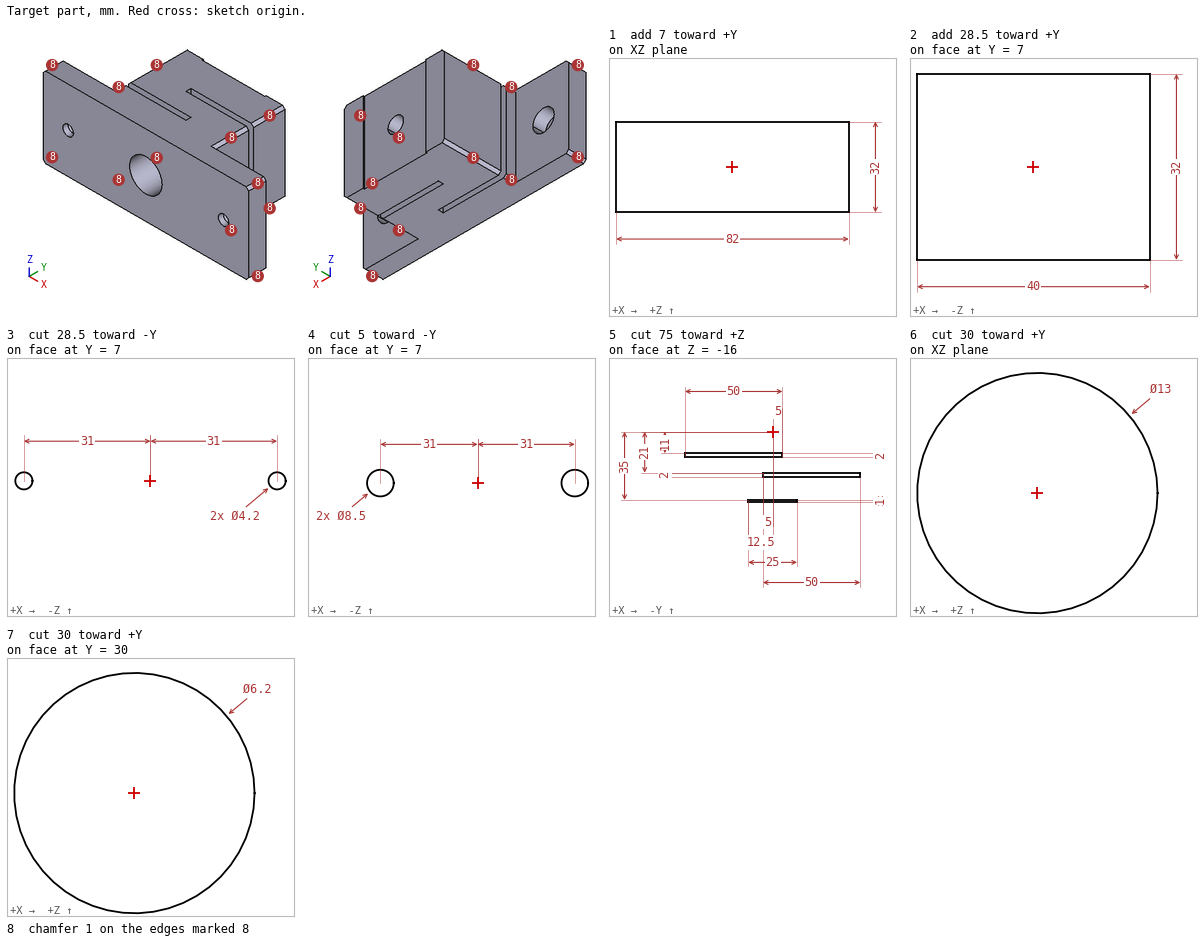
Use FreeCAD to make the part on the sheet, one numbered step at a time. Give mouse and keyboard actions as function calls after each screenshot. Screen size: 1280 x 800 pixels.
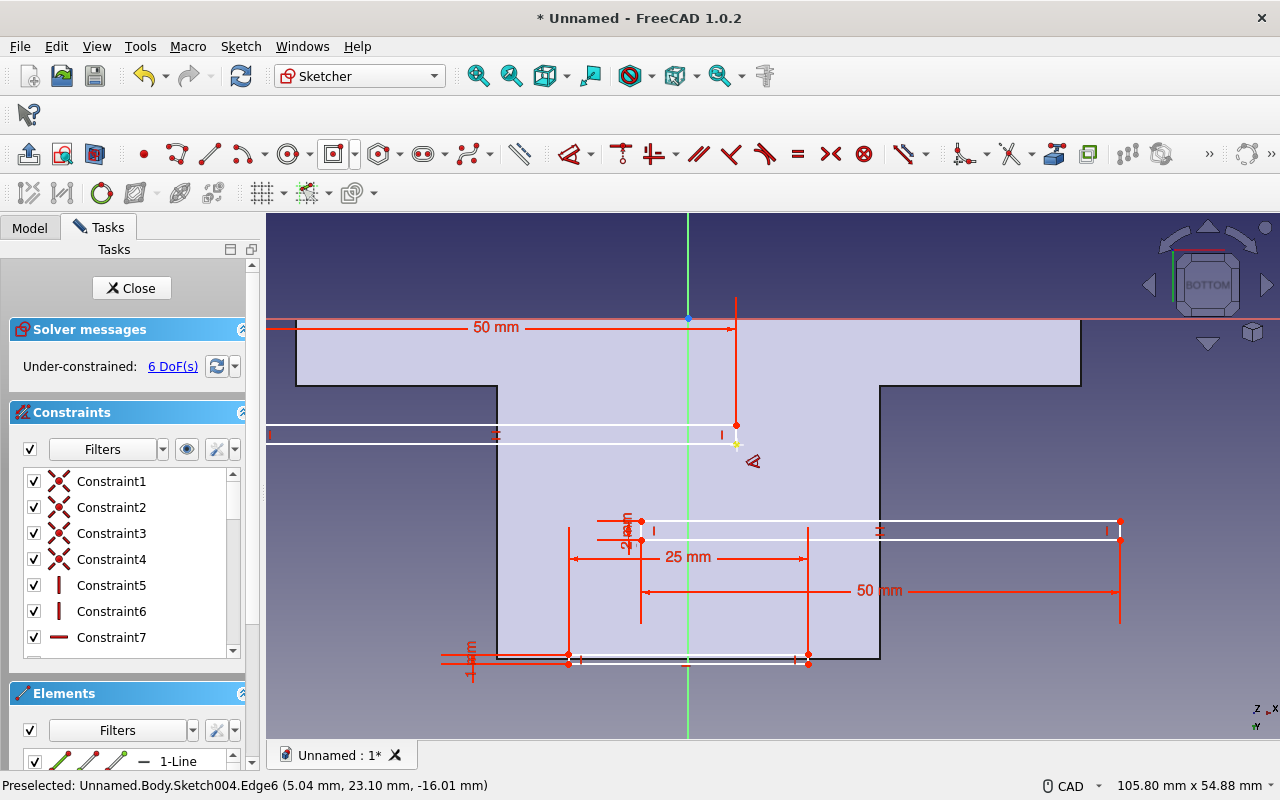
click(736, 444)
click(712, 285)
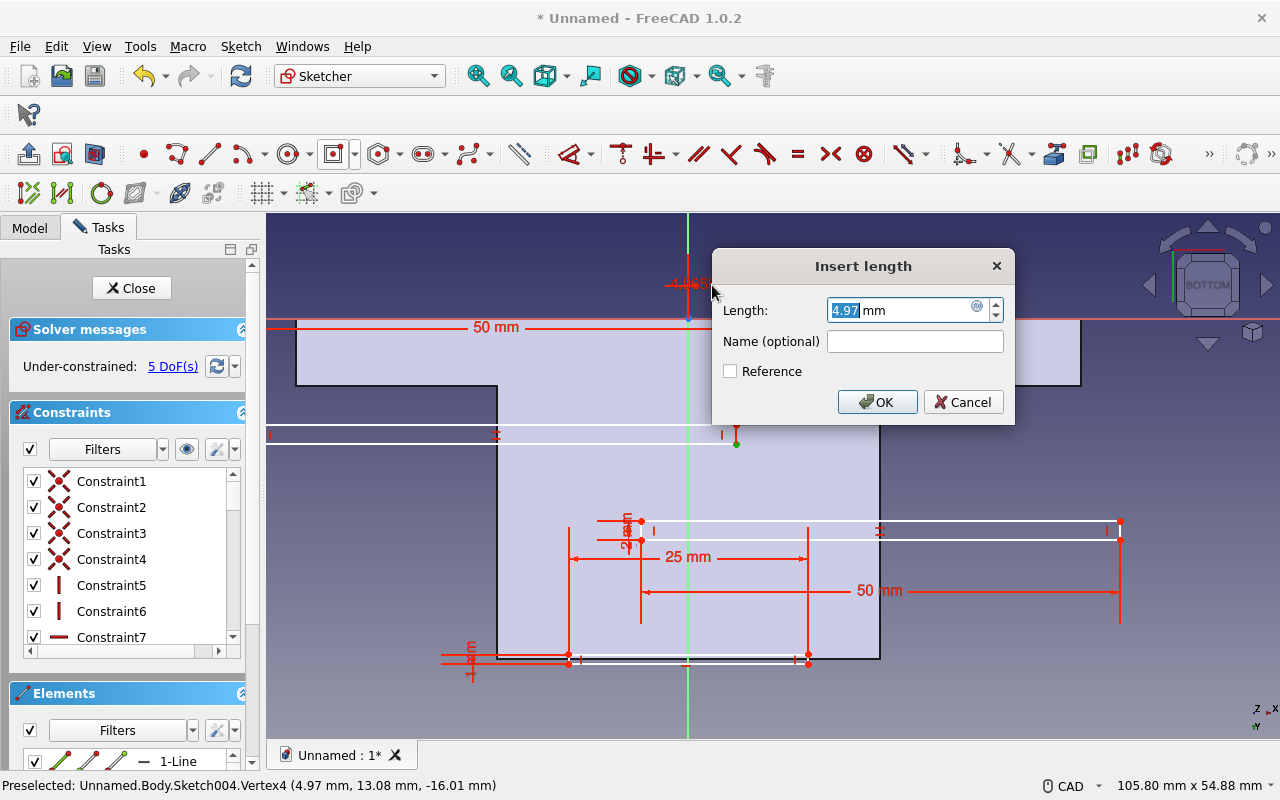
text(5)
key(Return)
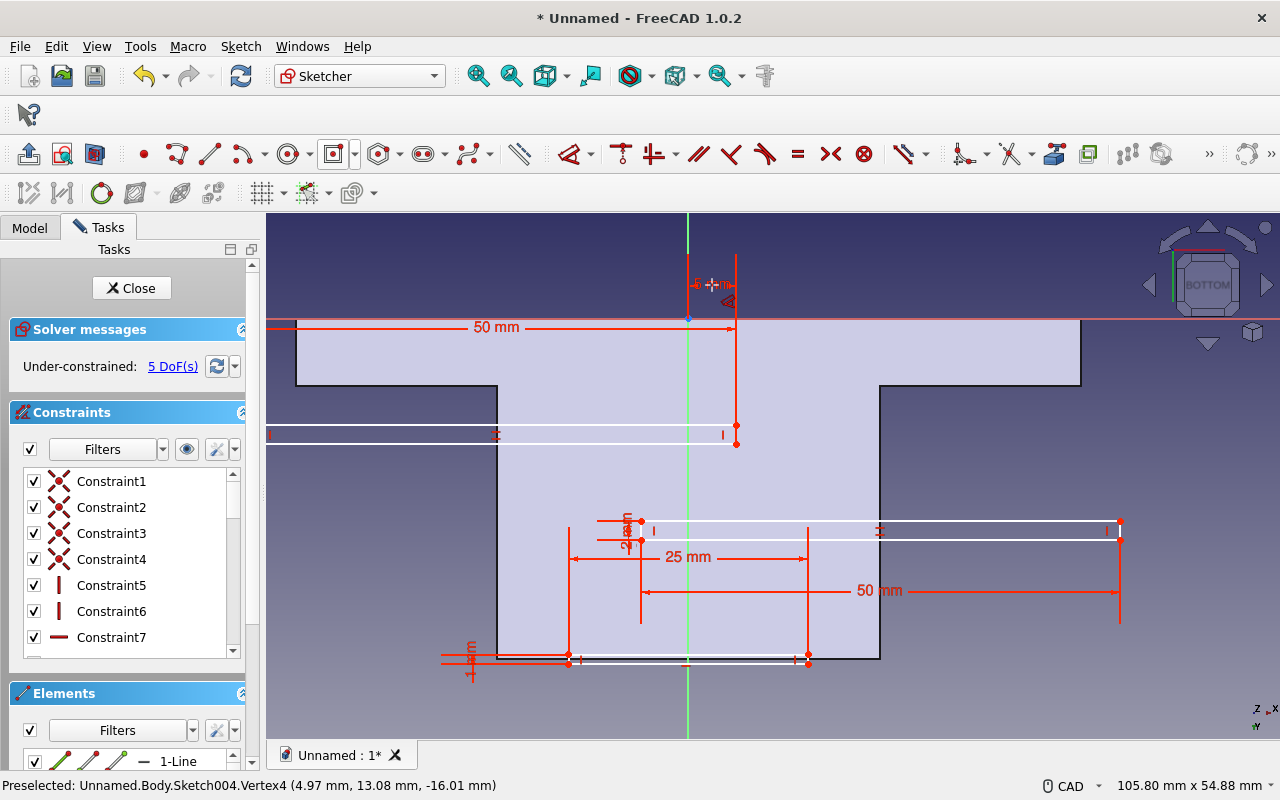
click(641, 521)
click(665, 555)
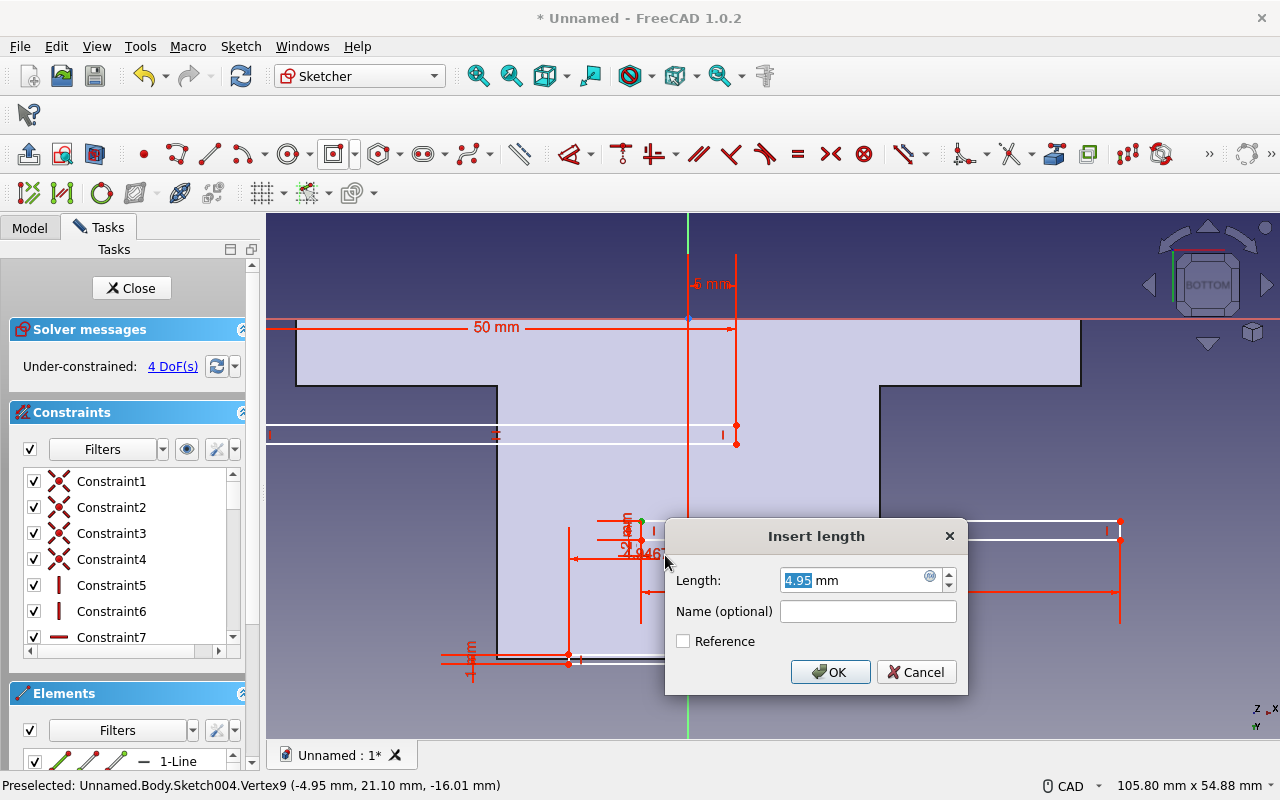
text(5)
key(Return)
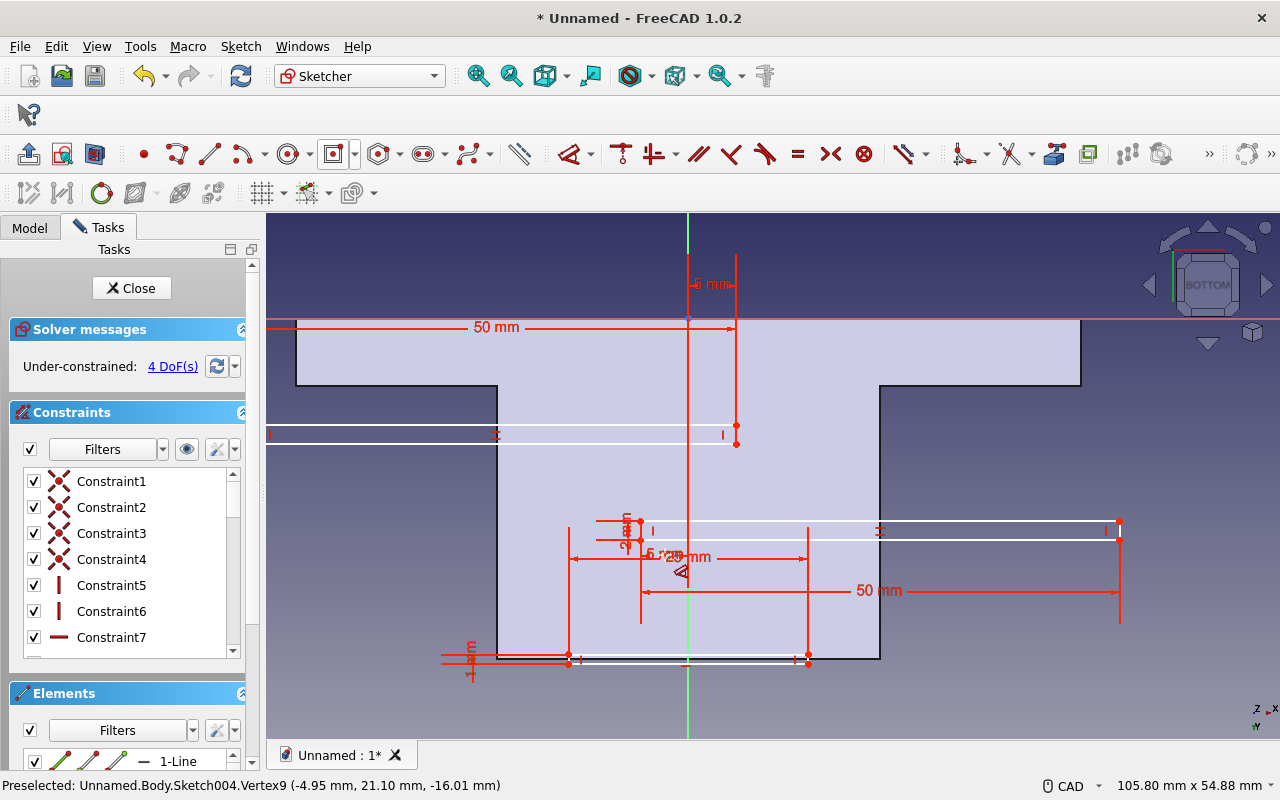
scroll(737, 445, down, 2)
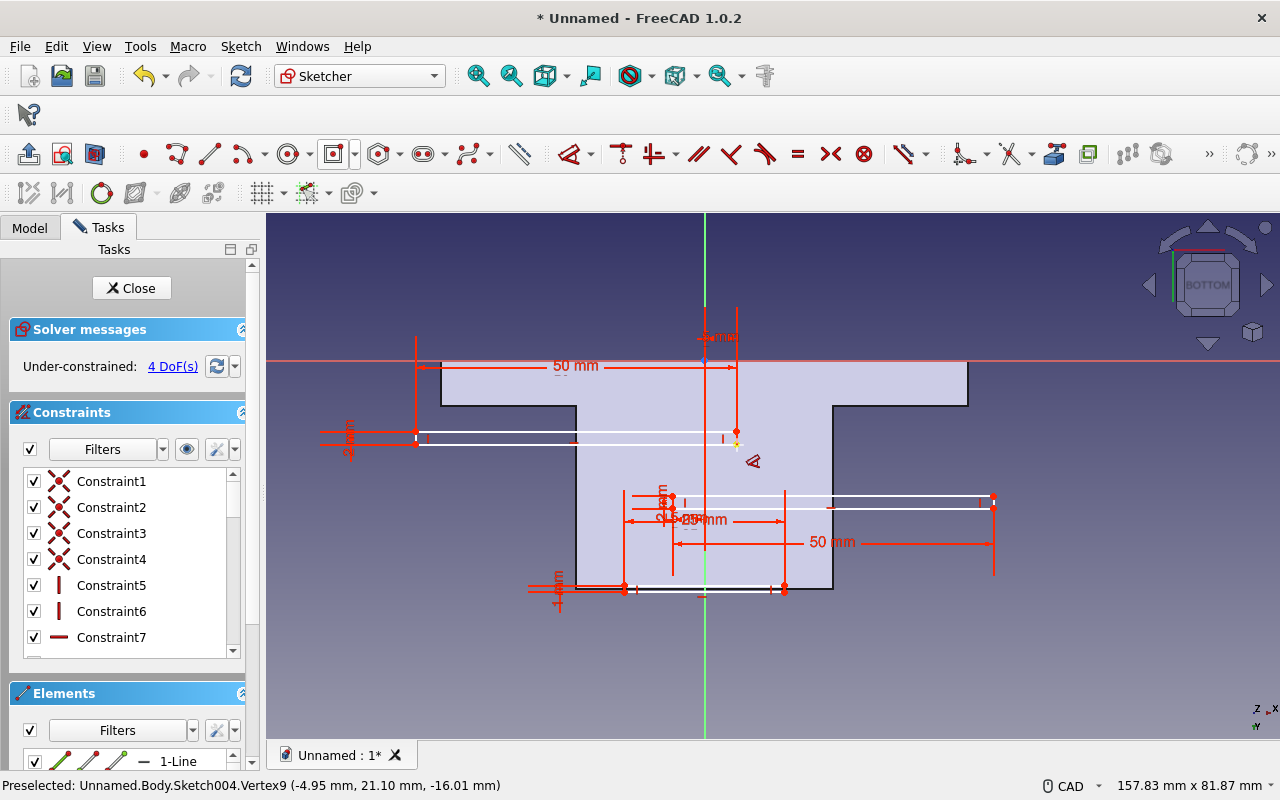
click(416, 432)
click(382, 396)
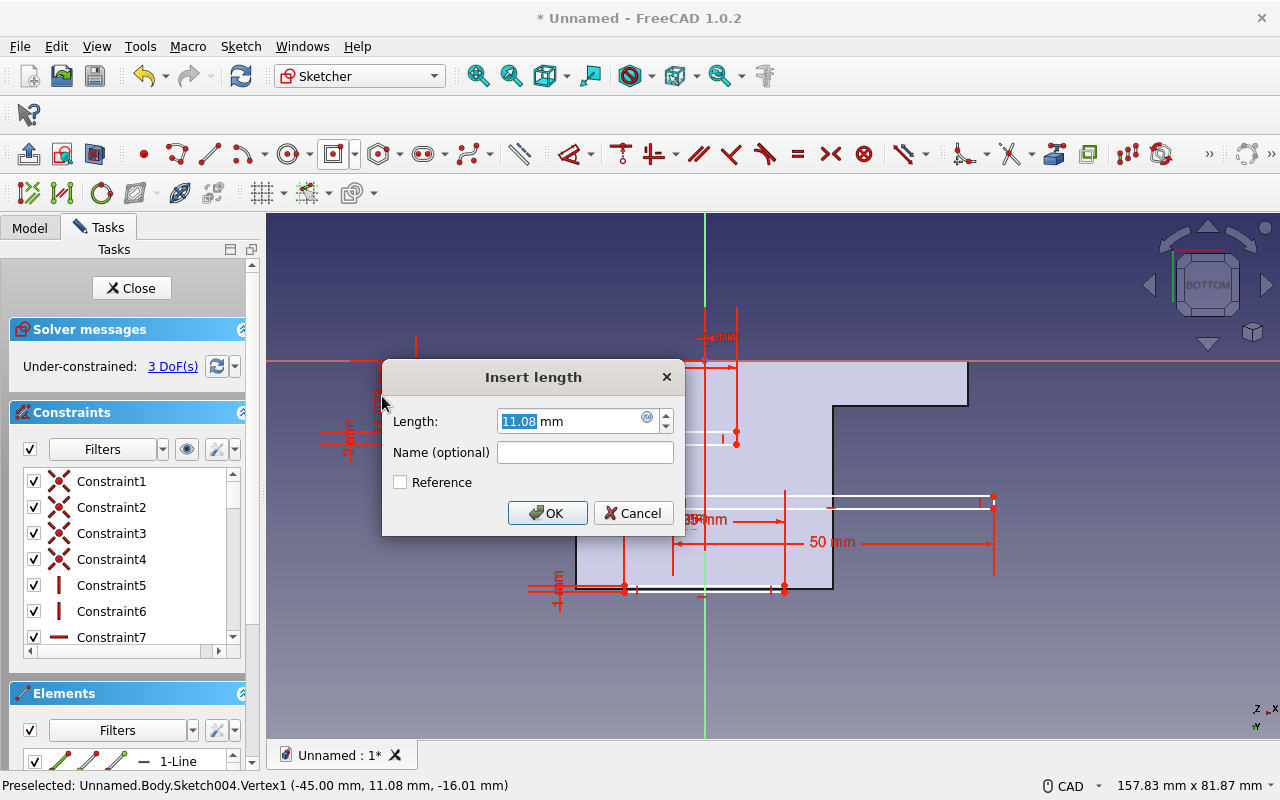
text(11)
key(Return)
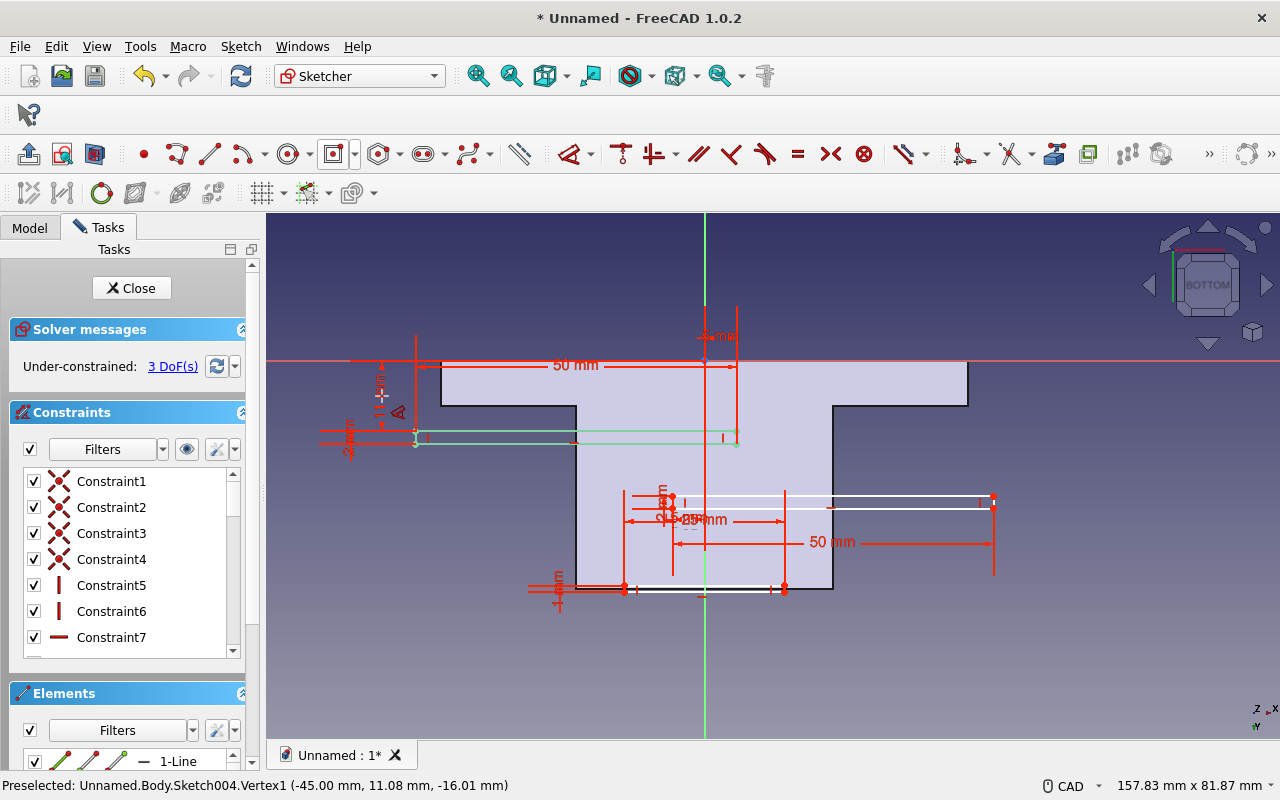
click(673, 496)
click(639, 397)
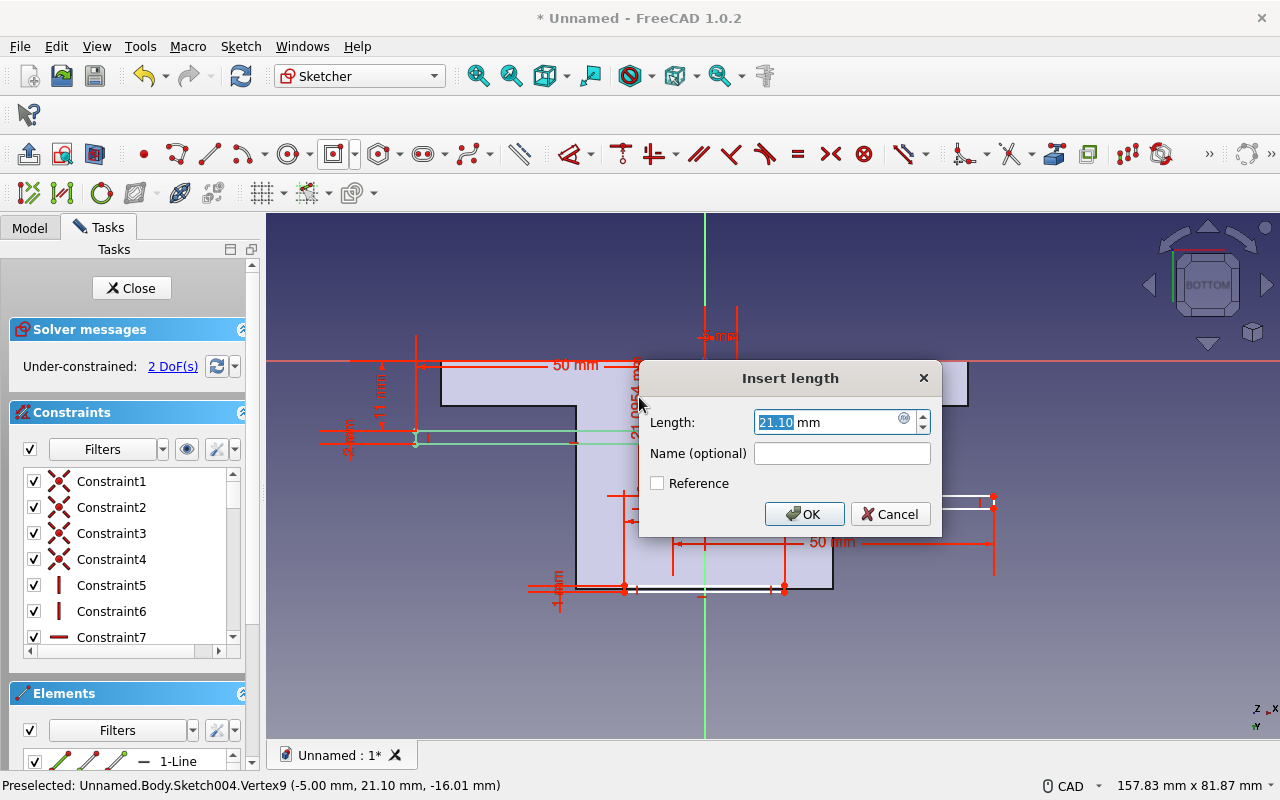
text(21)
key(Return)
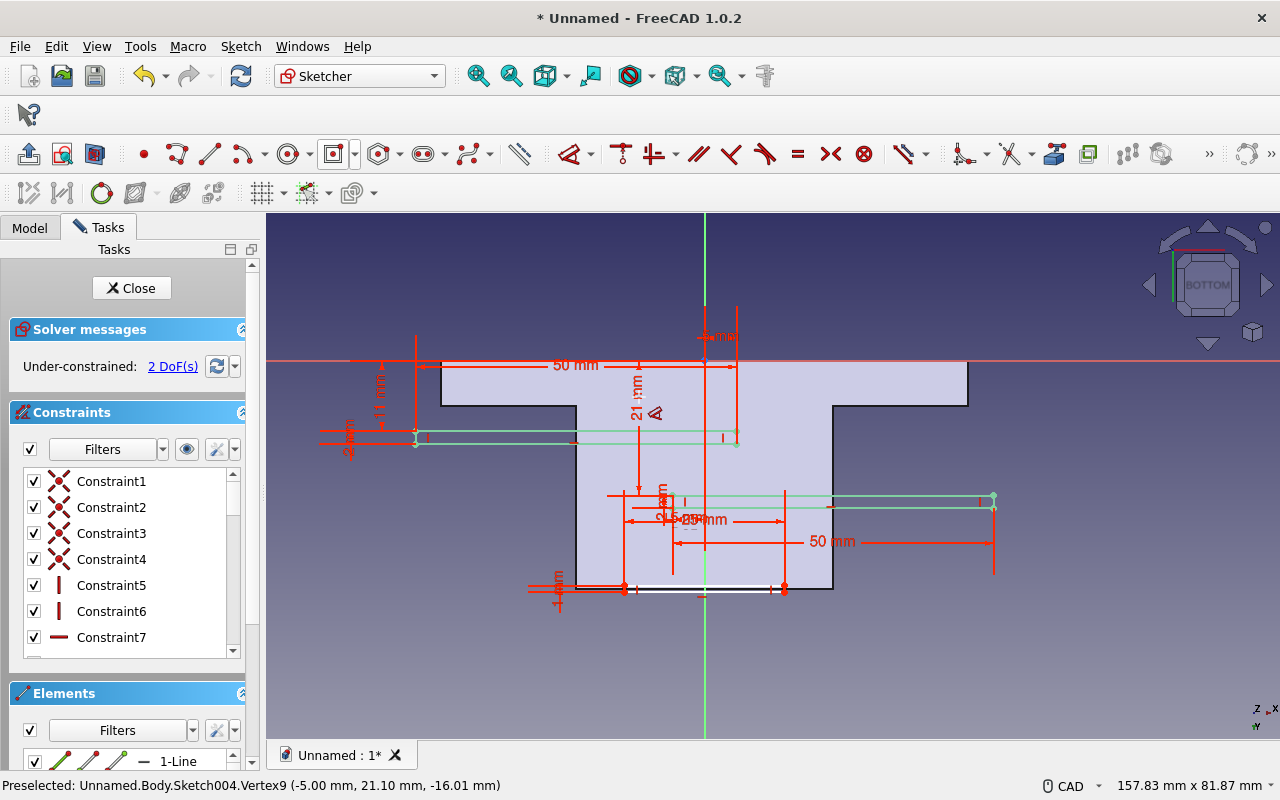
scroll(624, 586, up, 4)